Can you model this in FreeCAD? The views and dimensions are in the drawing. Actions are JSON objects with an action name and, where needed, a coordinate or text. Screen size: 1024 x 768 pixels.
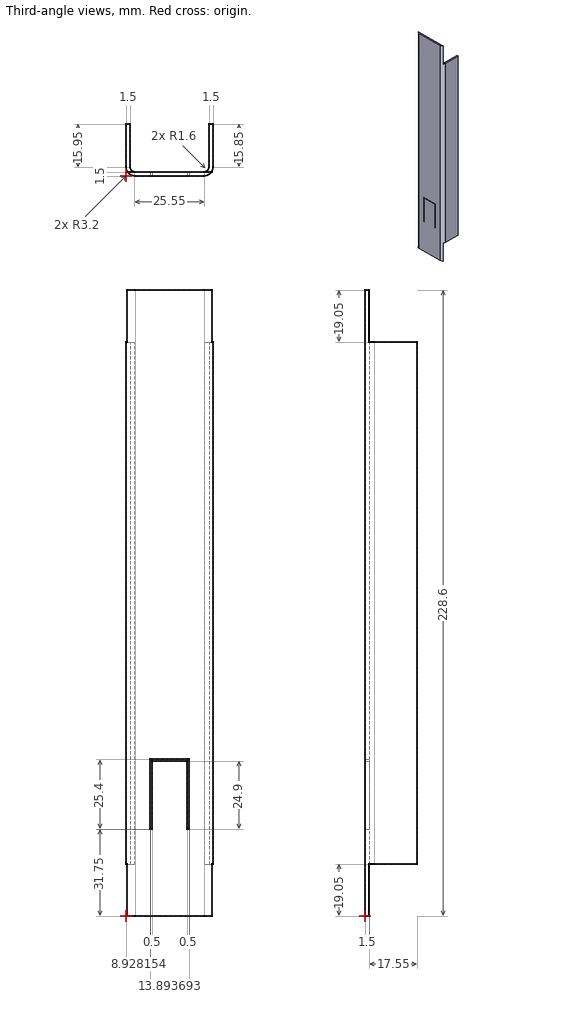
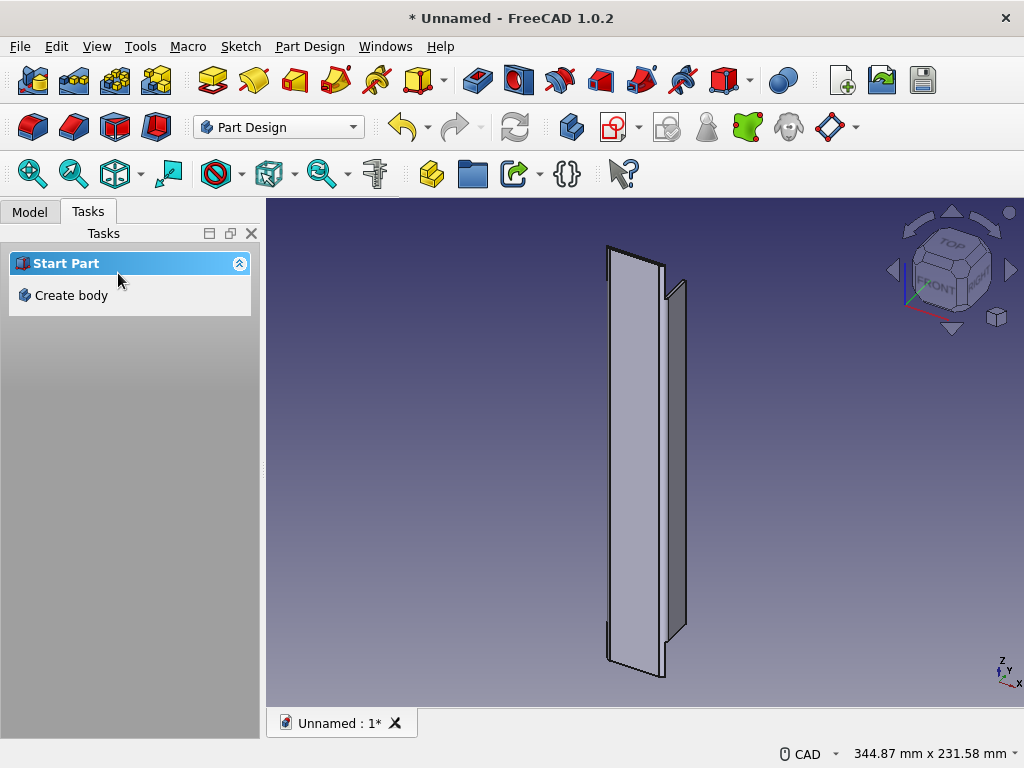
{"action": "left_click", "coordinate": [612, 128]}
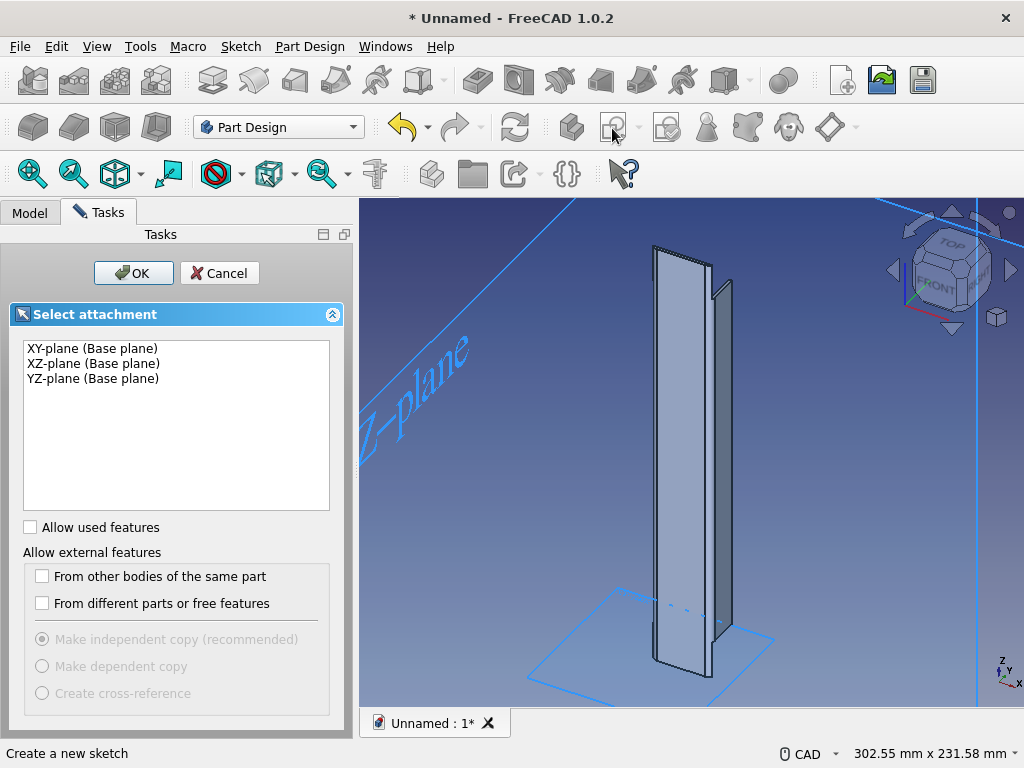
{"action": "left_click", "coordinate": [84, 364]}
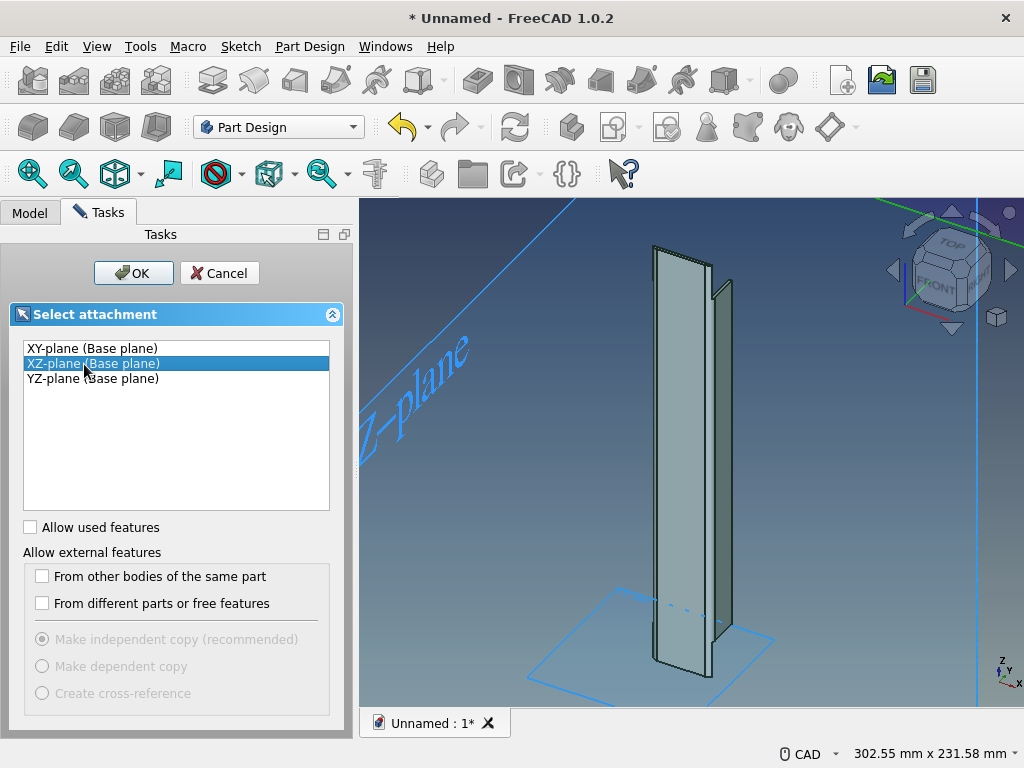
{"action": "left_click", "coordinate": [134, 273]}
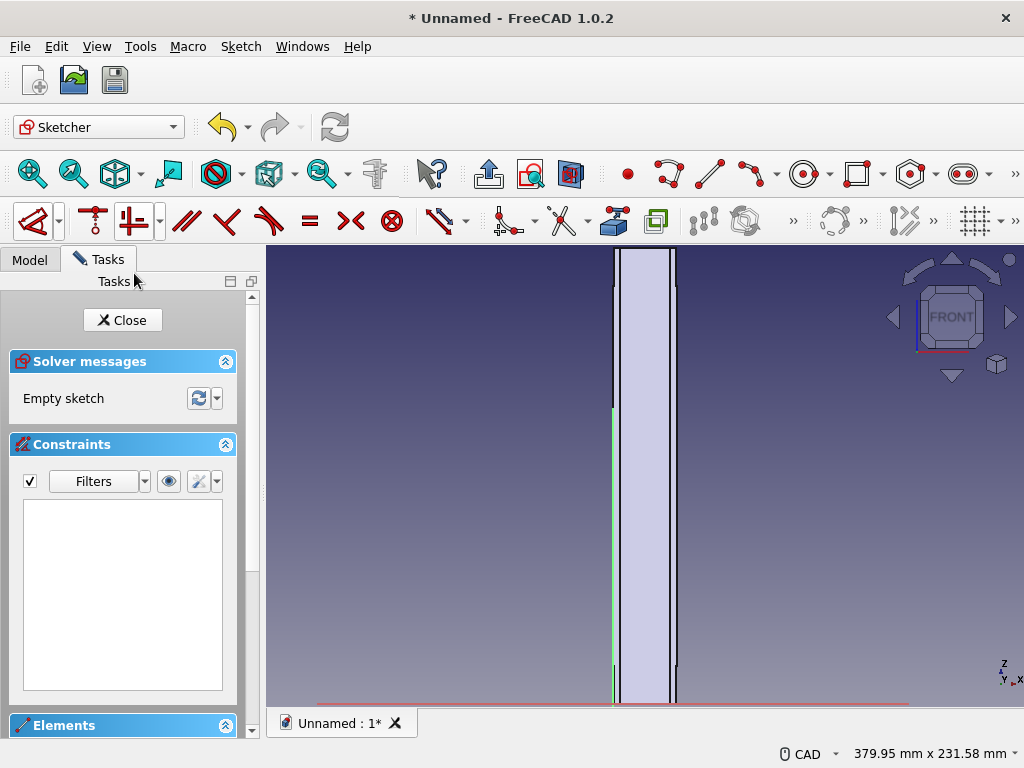
{"action": "scroll", "coordinate": [576, 476], "scroll_direction": "down", "scroll_amount": 5}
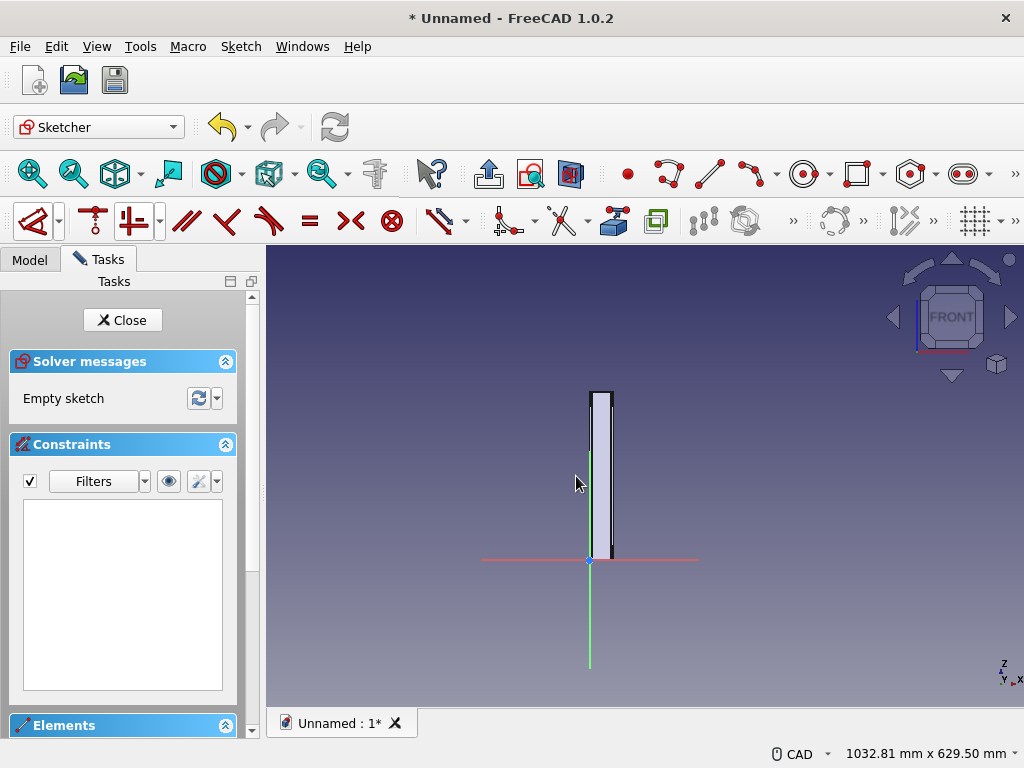
{"action": "scroll", "coordinate": [602, 549], "scroll_direction": "up", "scroll_amount": 10}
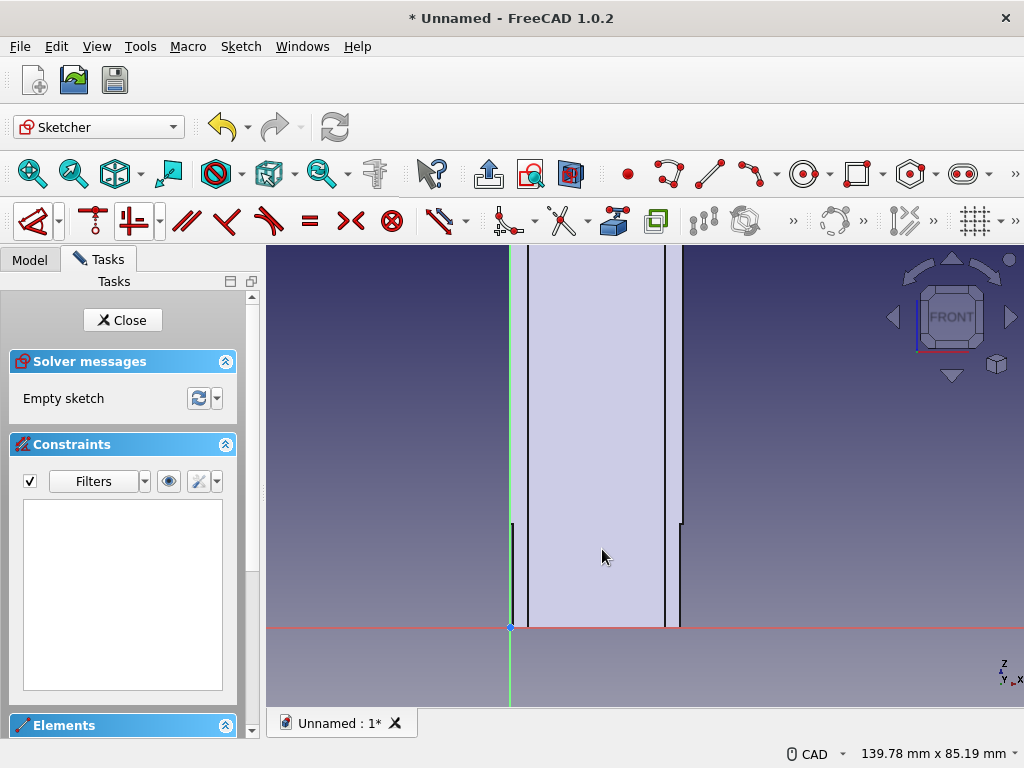
{"action": "left_click", "coordinate": [669, 174]}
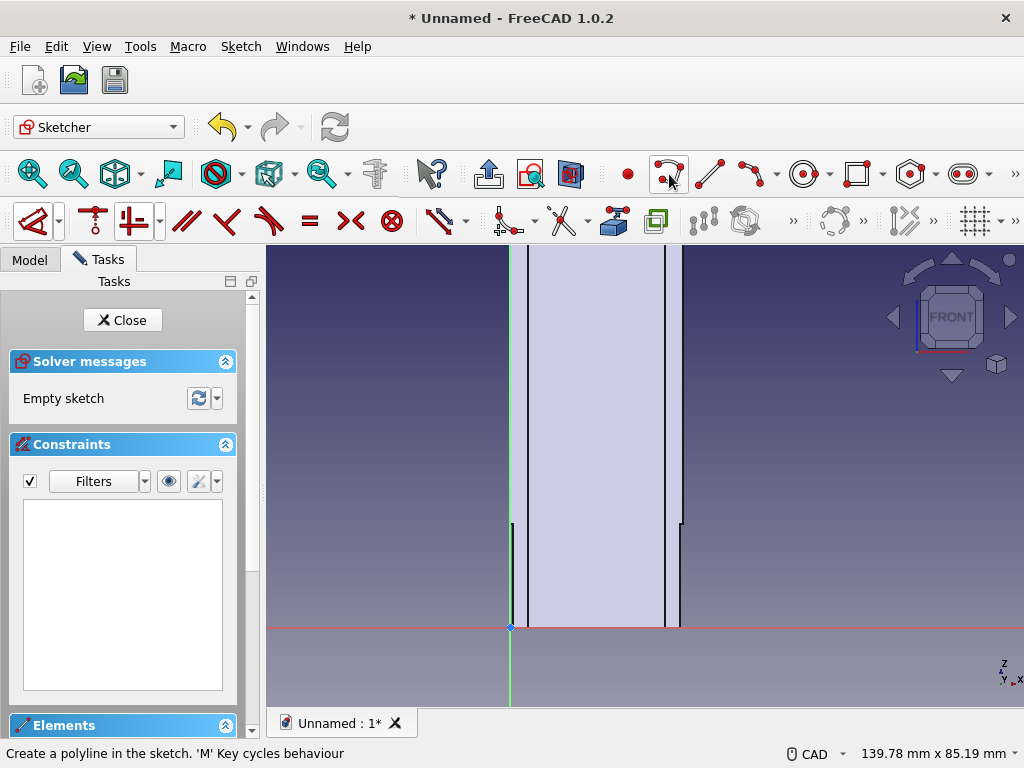
{"action": "left_click", "coordinate": [559, 455]}
{"action": "left_click", "coordinate": [559, 318]}
{"action": "left_click", "coordinate": [634, 318]}
{"action": "left_click", "coordinate": [634, 455]}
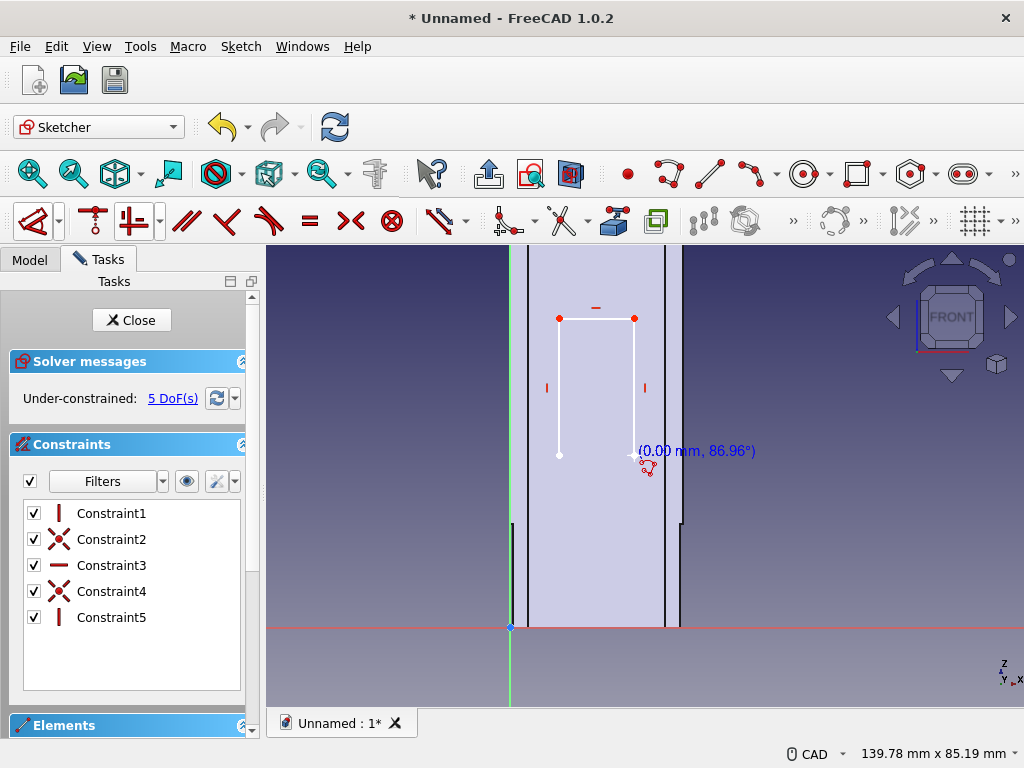
{"action": "scroll", "coordinate": [631, 455], "scroll_direction": "up", "scroll_amount": 9}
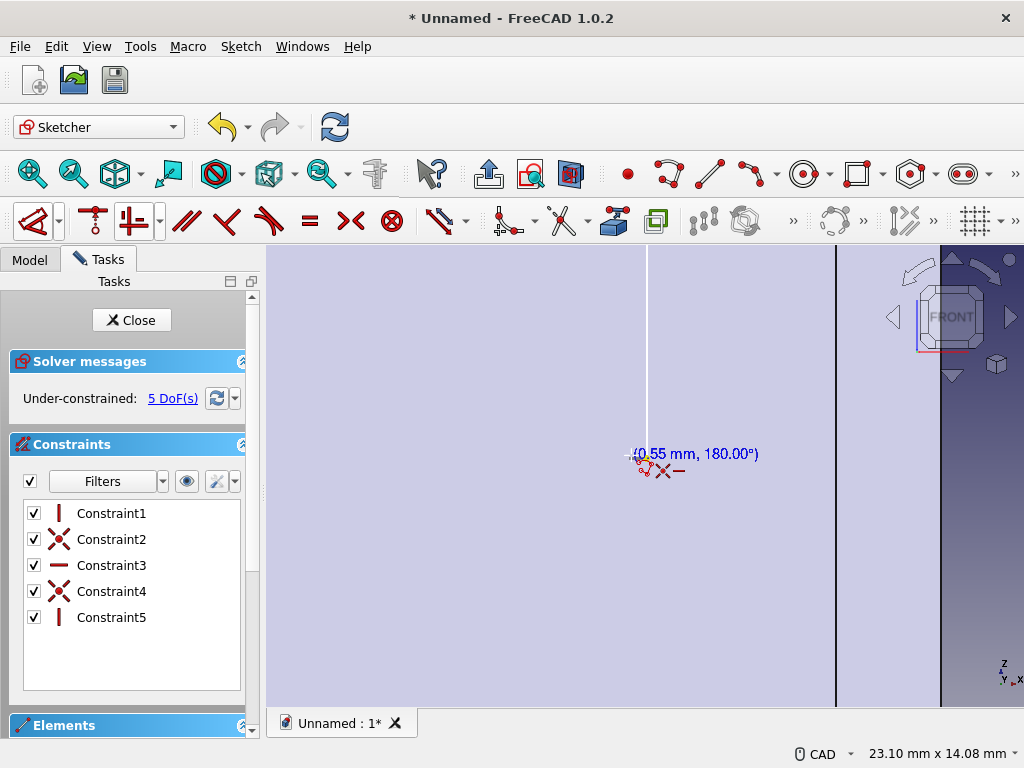
{"action": "left_click", "coordinate": [631, 453]}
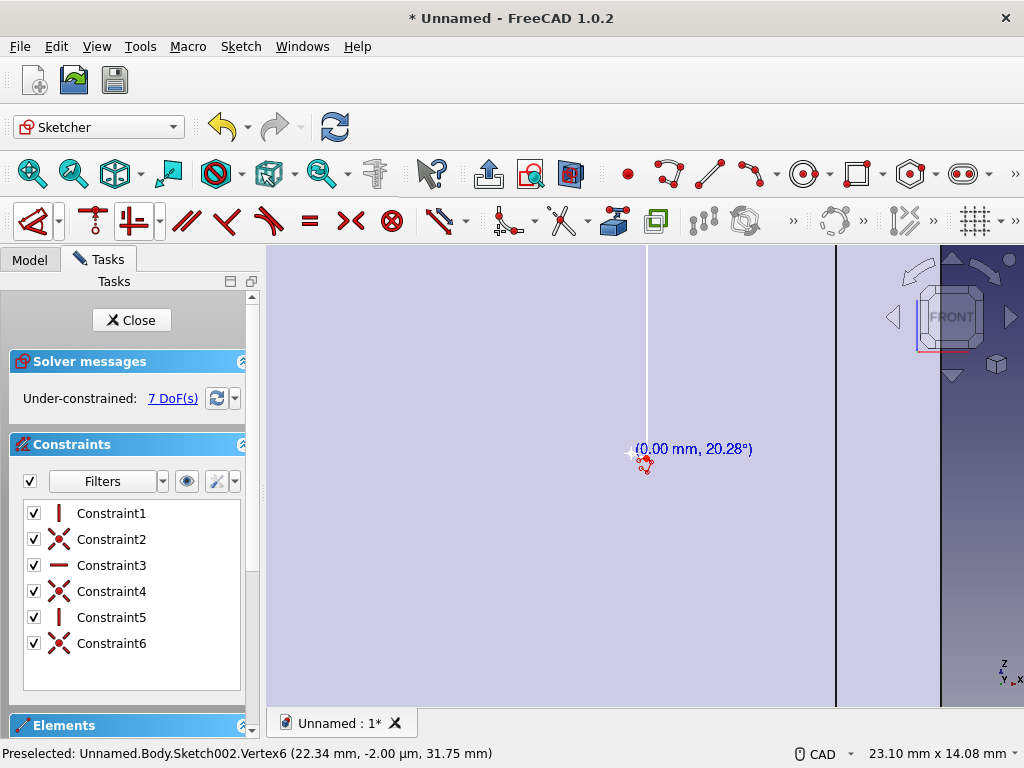
{"action": "scroll", "coordinate": [636, 460], "scroll_direction": "down", "scroll_amount": 9}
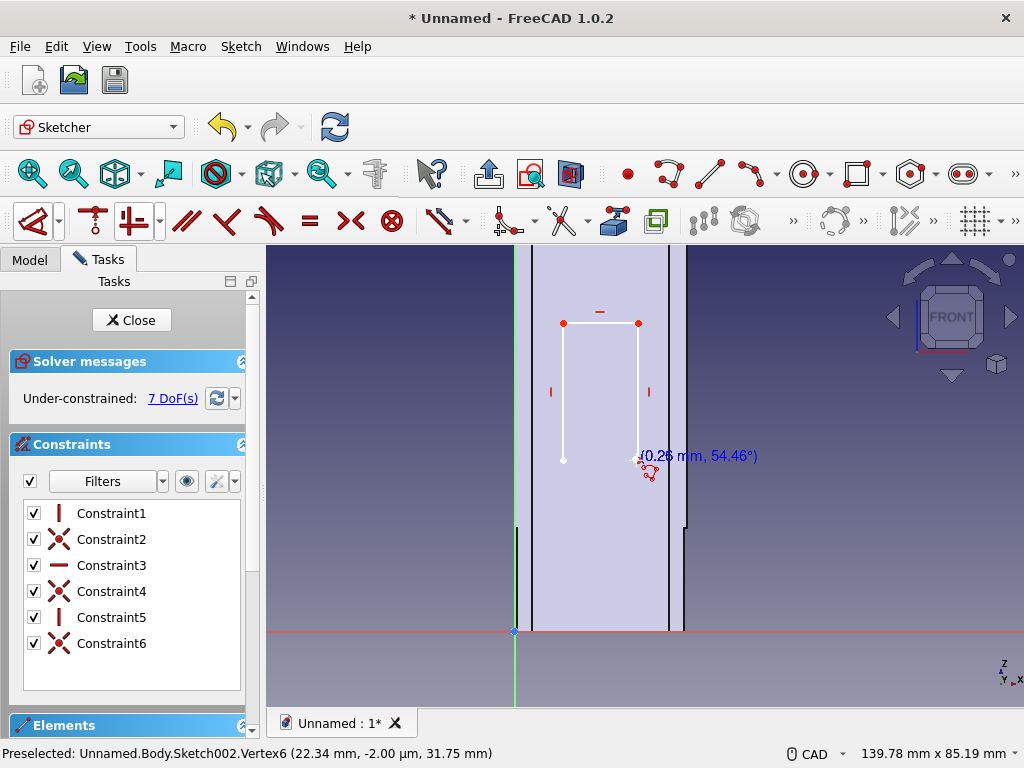
{"action": "scroll", "coordinate": [636, 325], "scroll_direction": "up", "scroll_amount": 9}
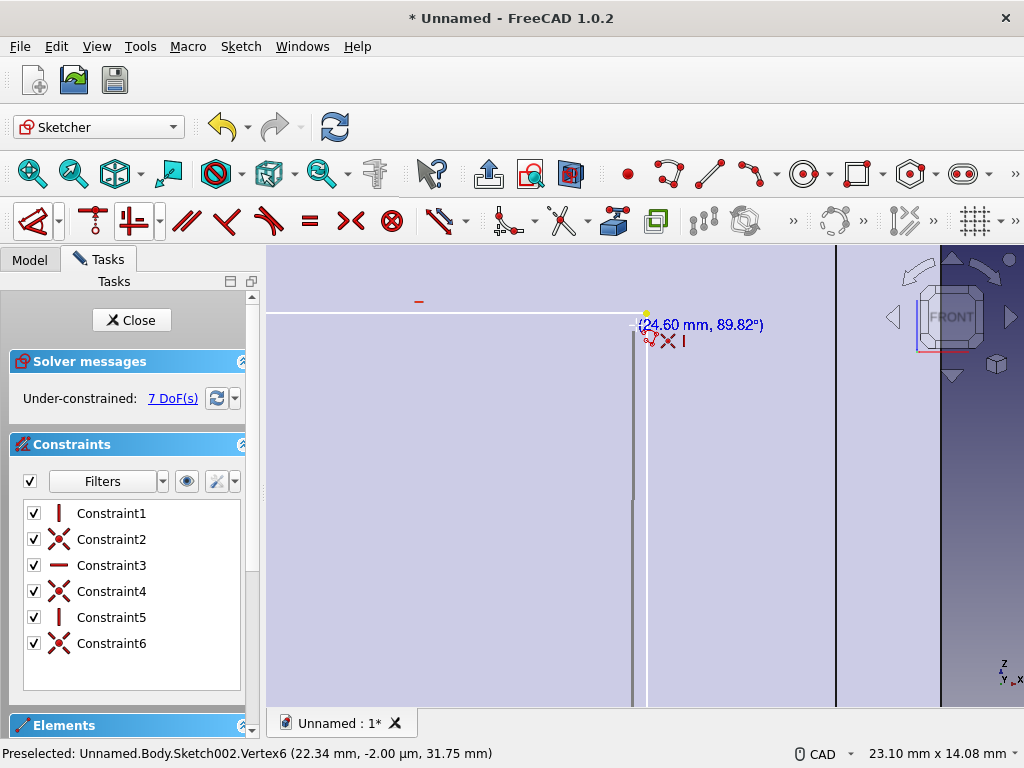
{"action": "left_click", "coordinate": [631, 321]}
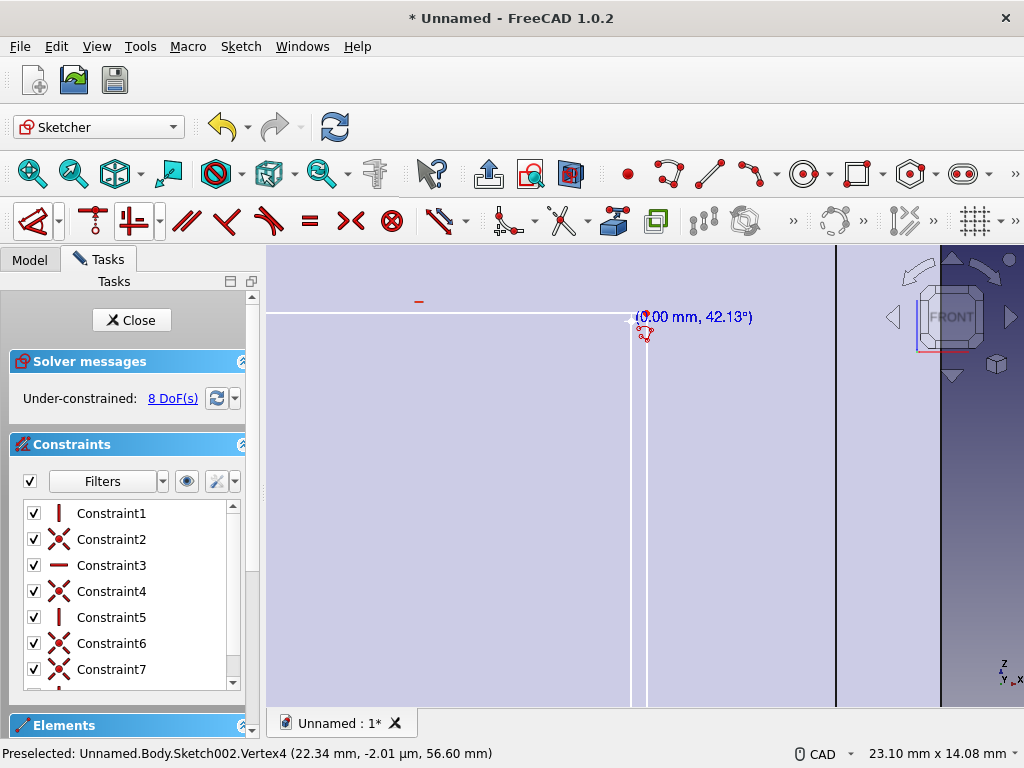
{"action": "scroll", "coordinate": [636, 324], "scroll_direction": "down", "scroll_amount": 9}